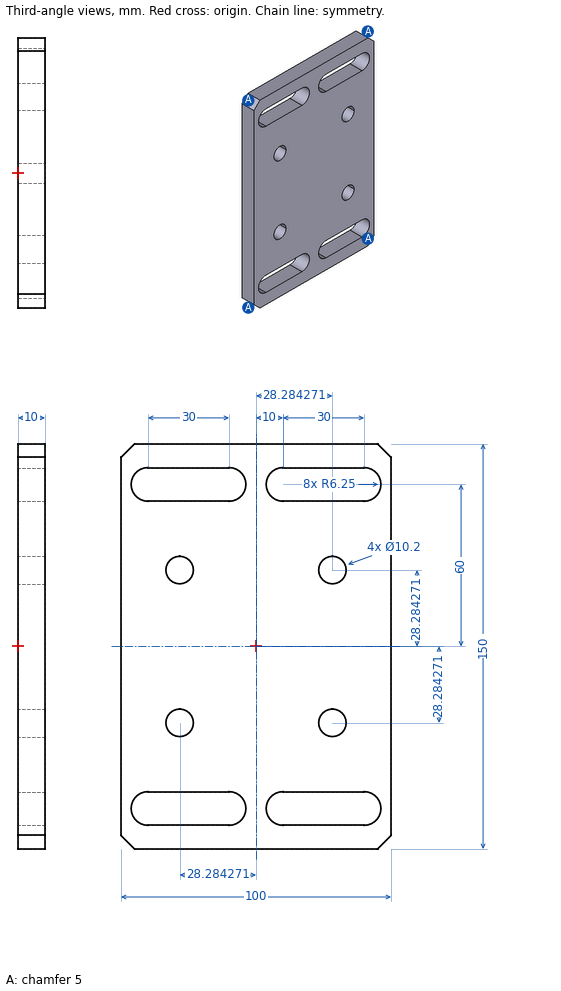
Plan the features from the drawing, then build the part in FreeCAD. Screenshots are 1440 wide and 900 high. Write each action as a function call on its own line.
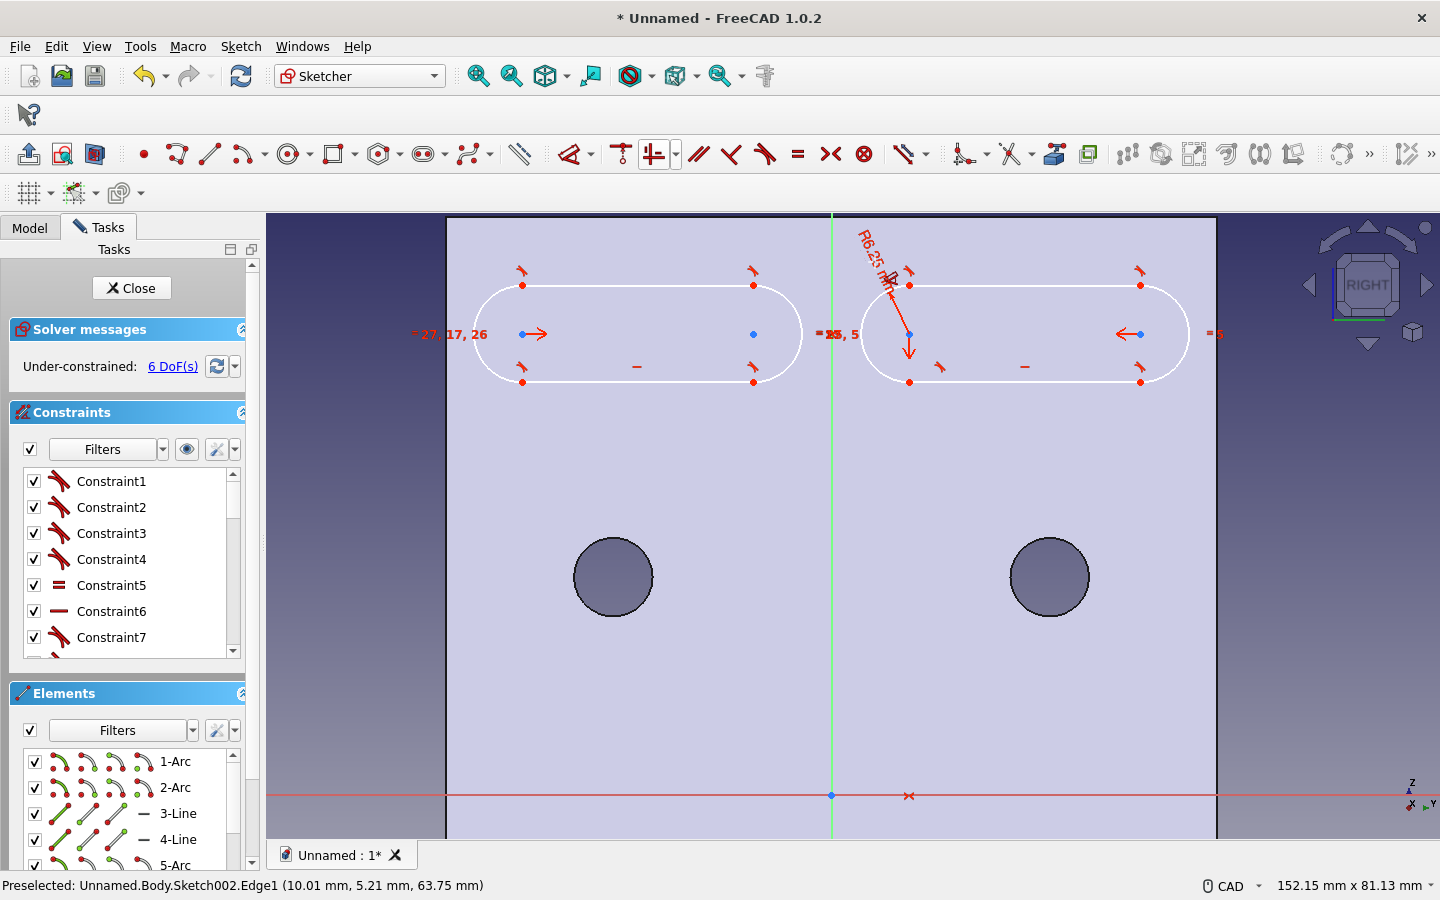
click(979, 286)
click(1025, 252)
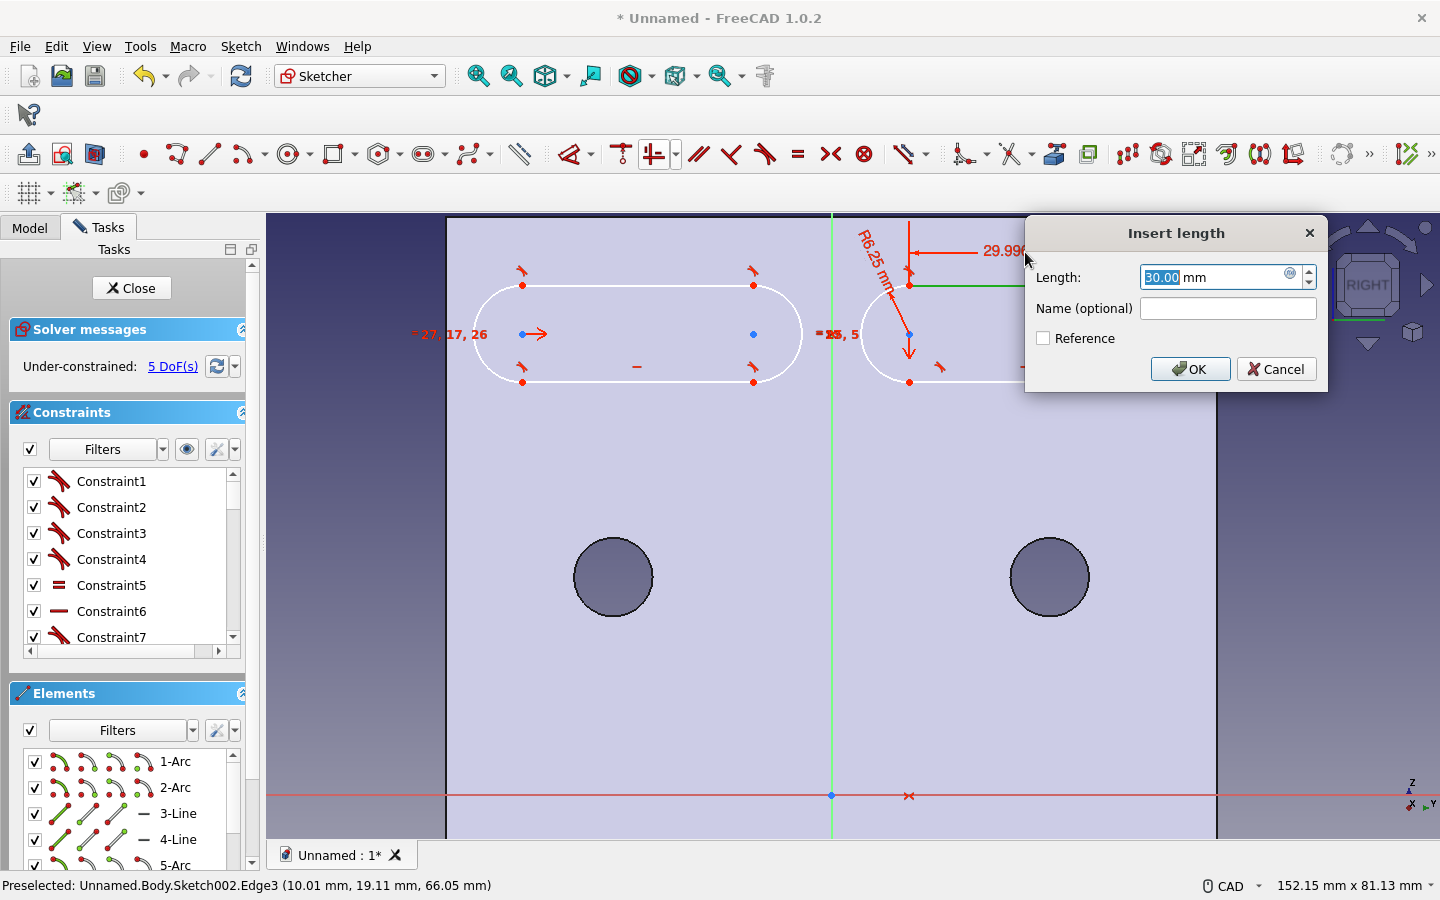
text(30)
key(Return)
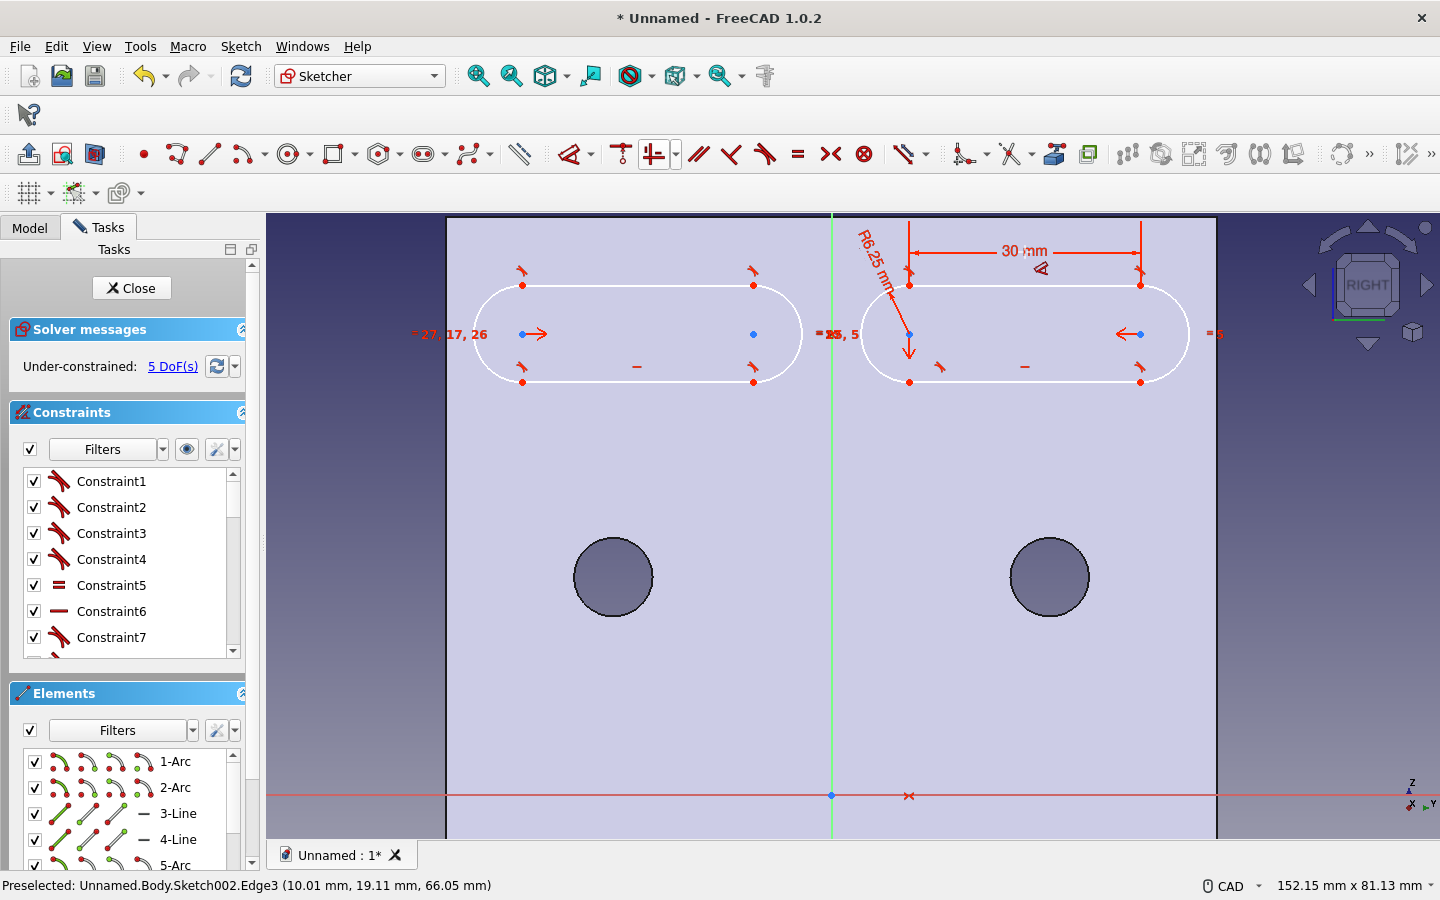
scroll(757, 369, down, 5)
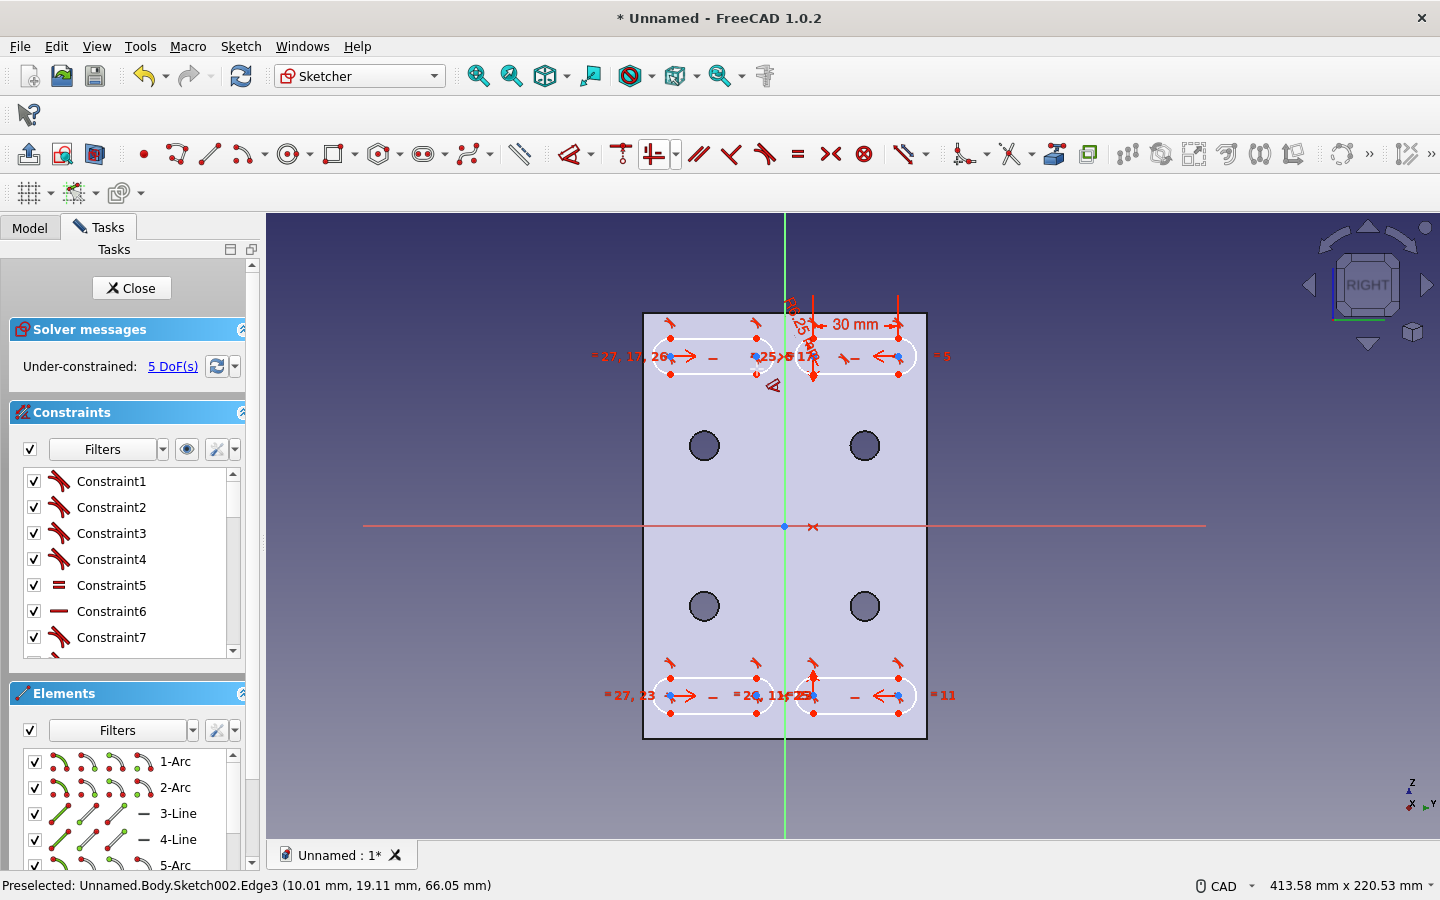
click(839, 678)
click(856, 644)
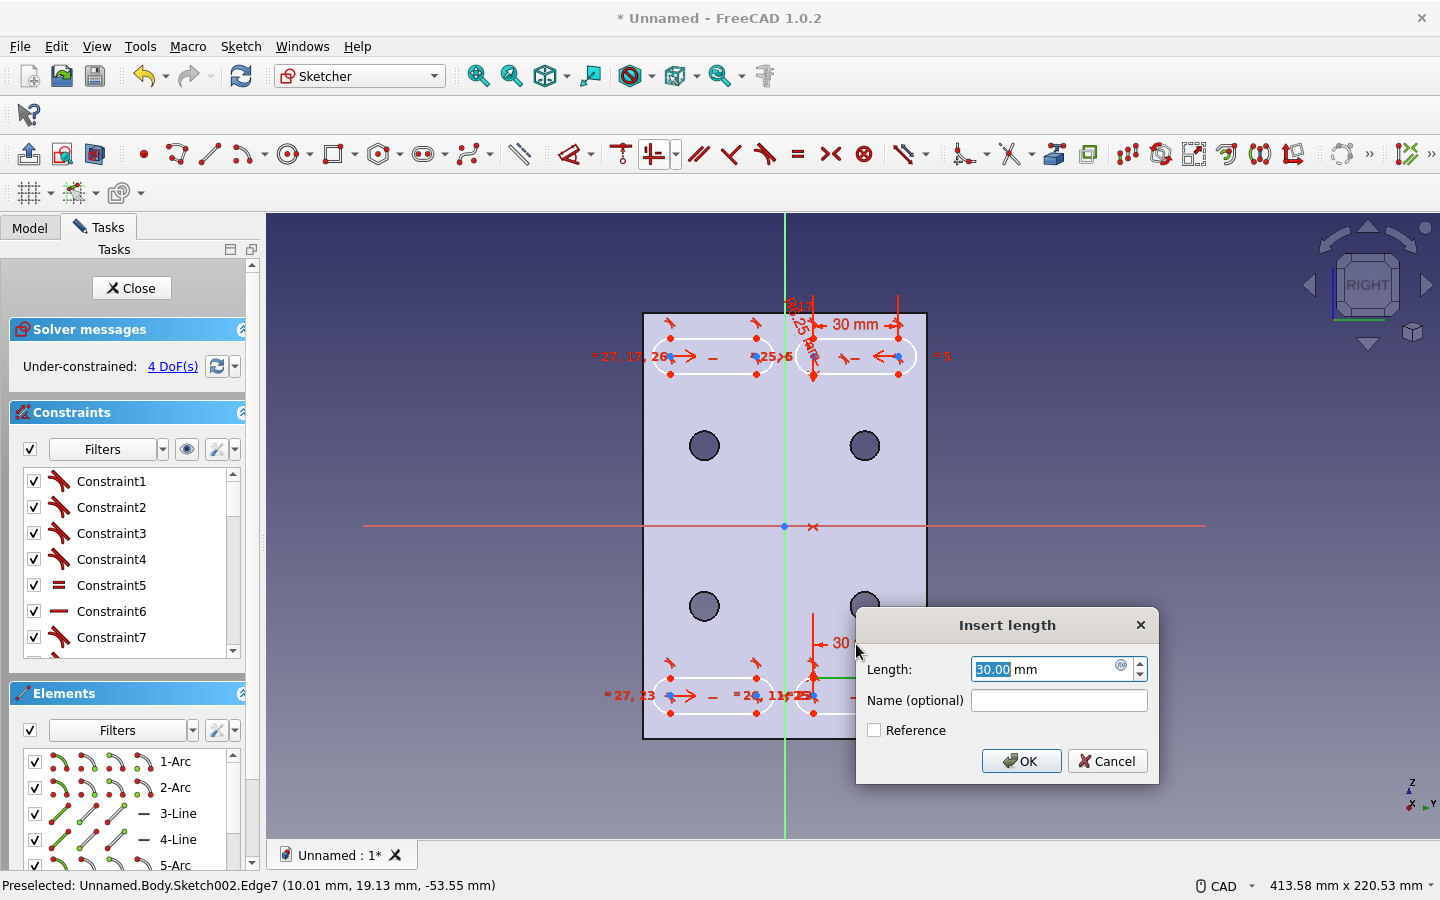
text(30)
key(Return)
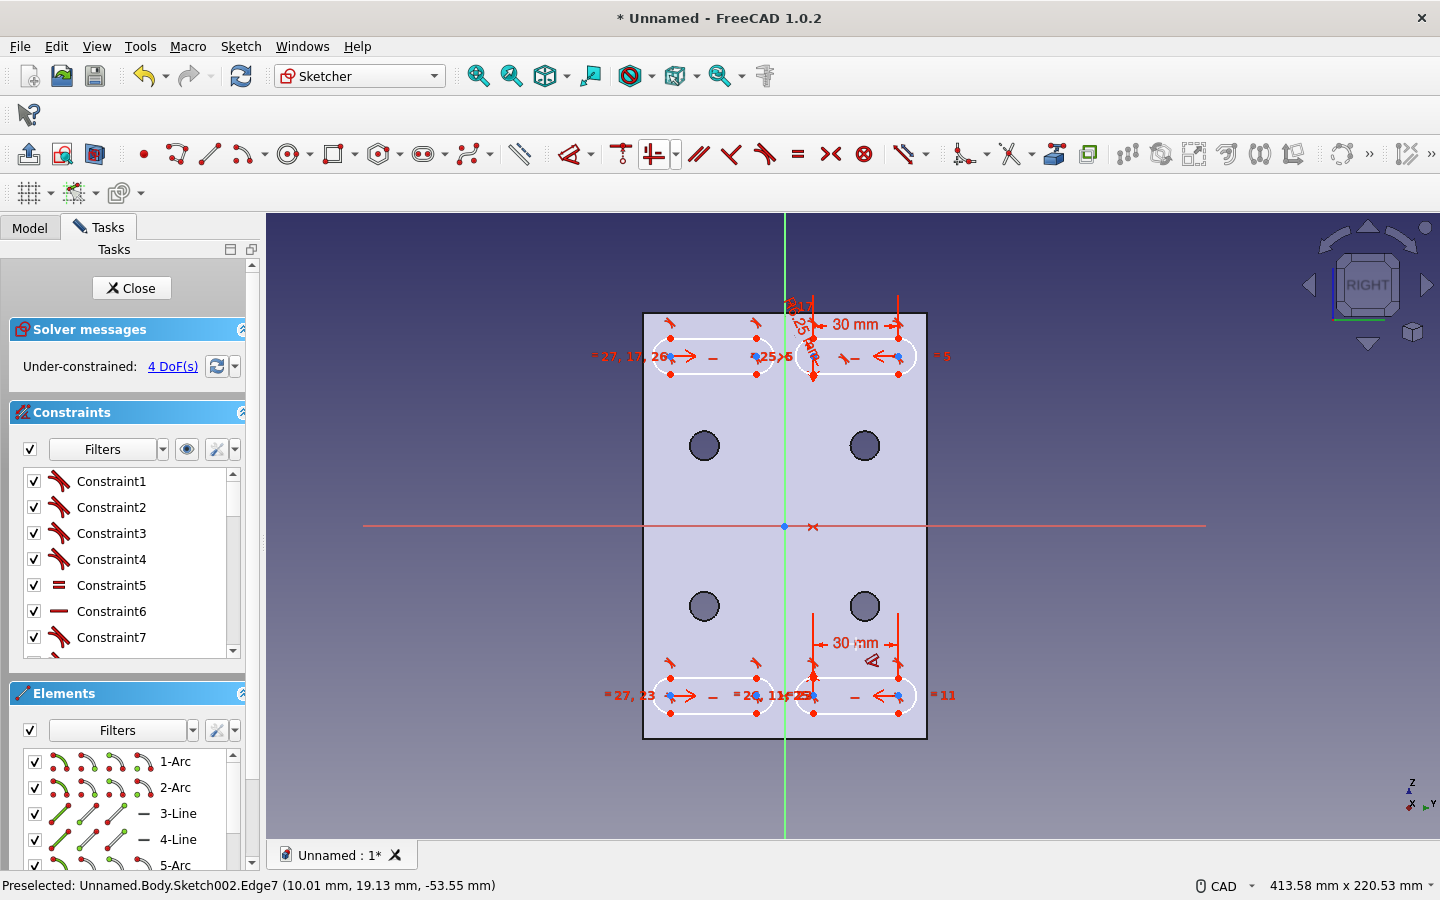
click(696, 339)
click(713, 305)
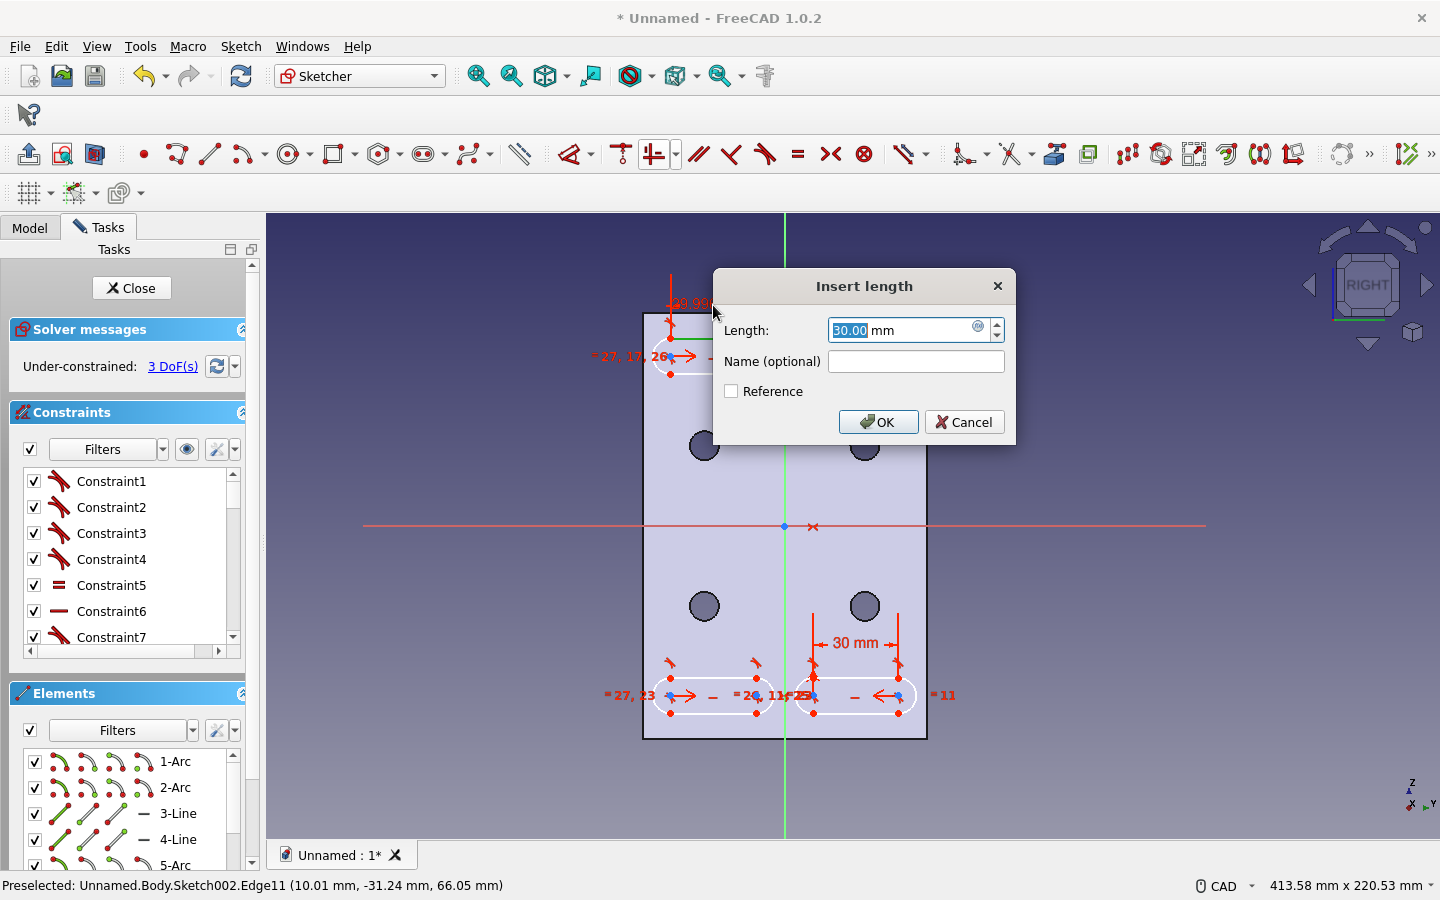
text(30)
key(Return)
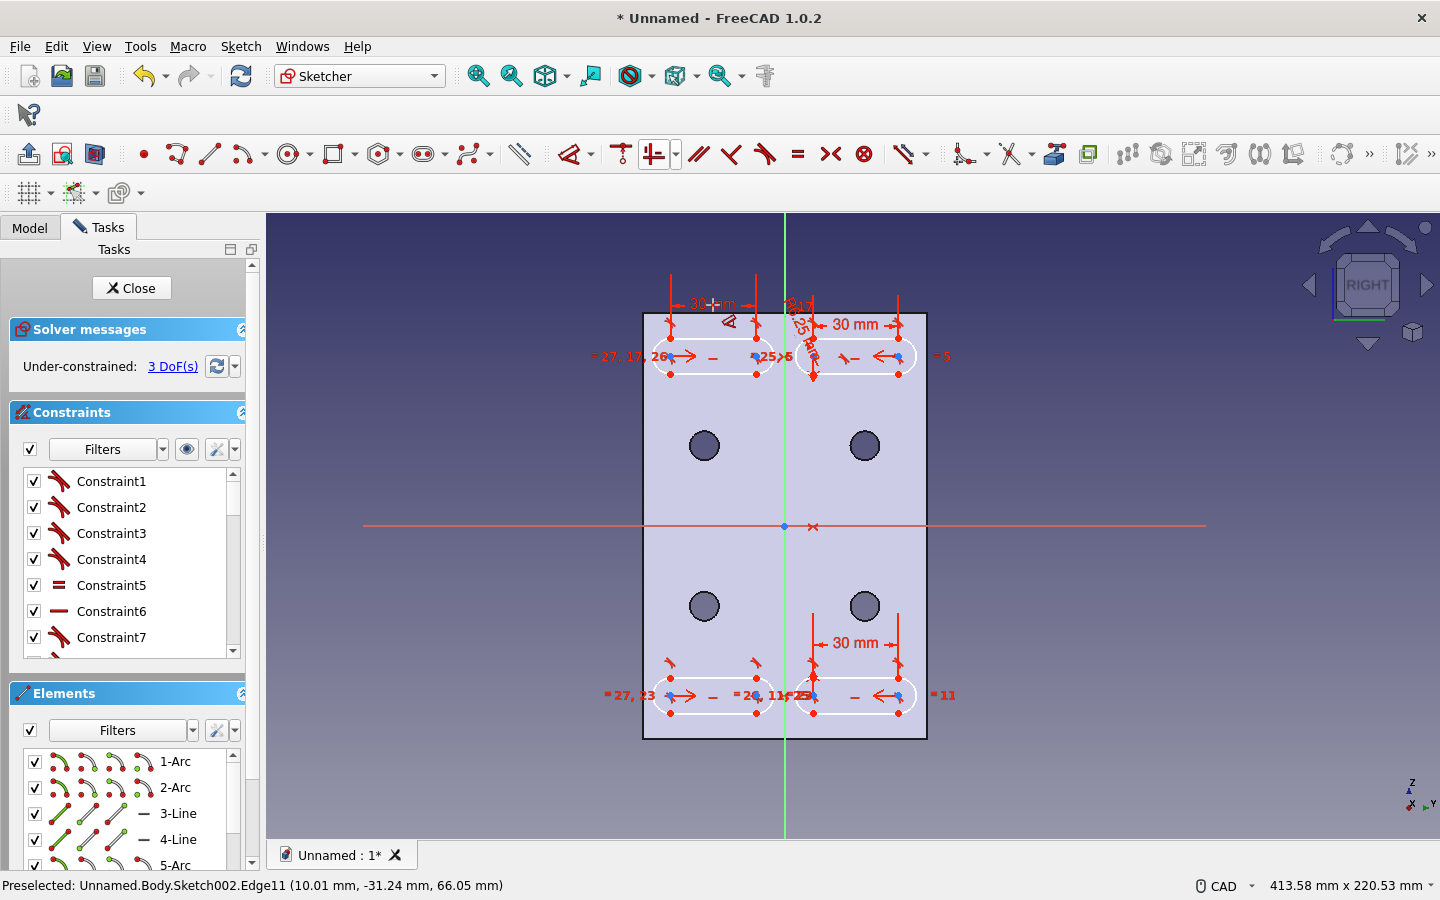
click(696, 678)
click(713, 644)